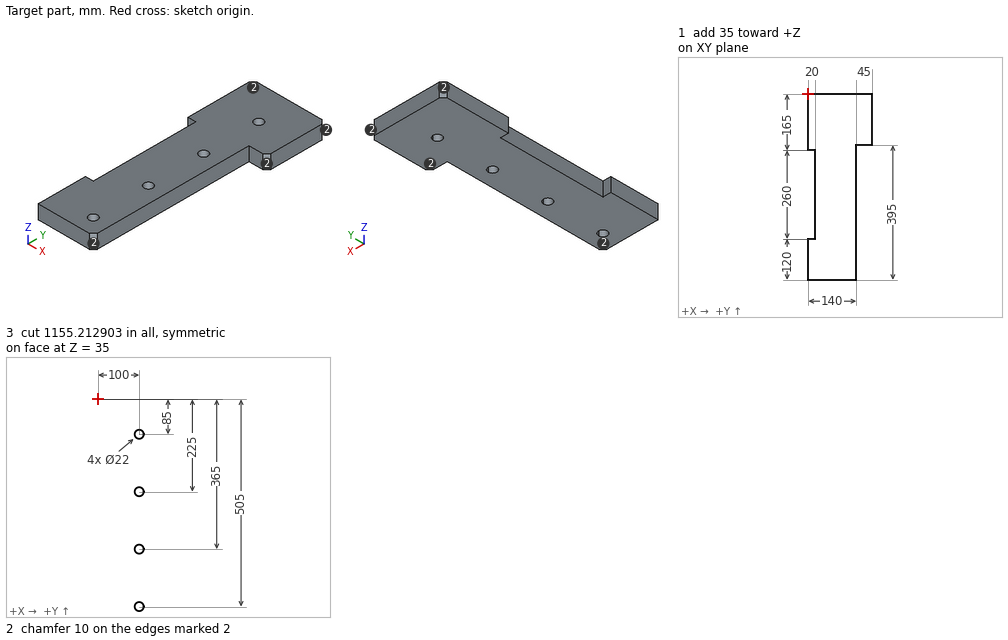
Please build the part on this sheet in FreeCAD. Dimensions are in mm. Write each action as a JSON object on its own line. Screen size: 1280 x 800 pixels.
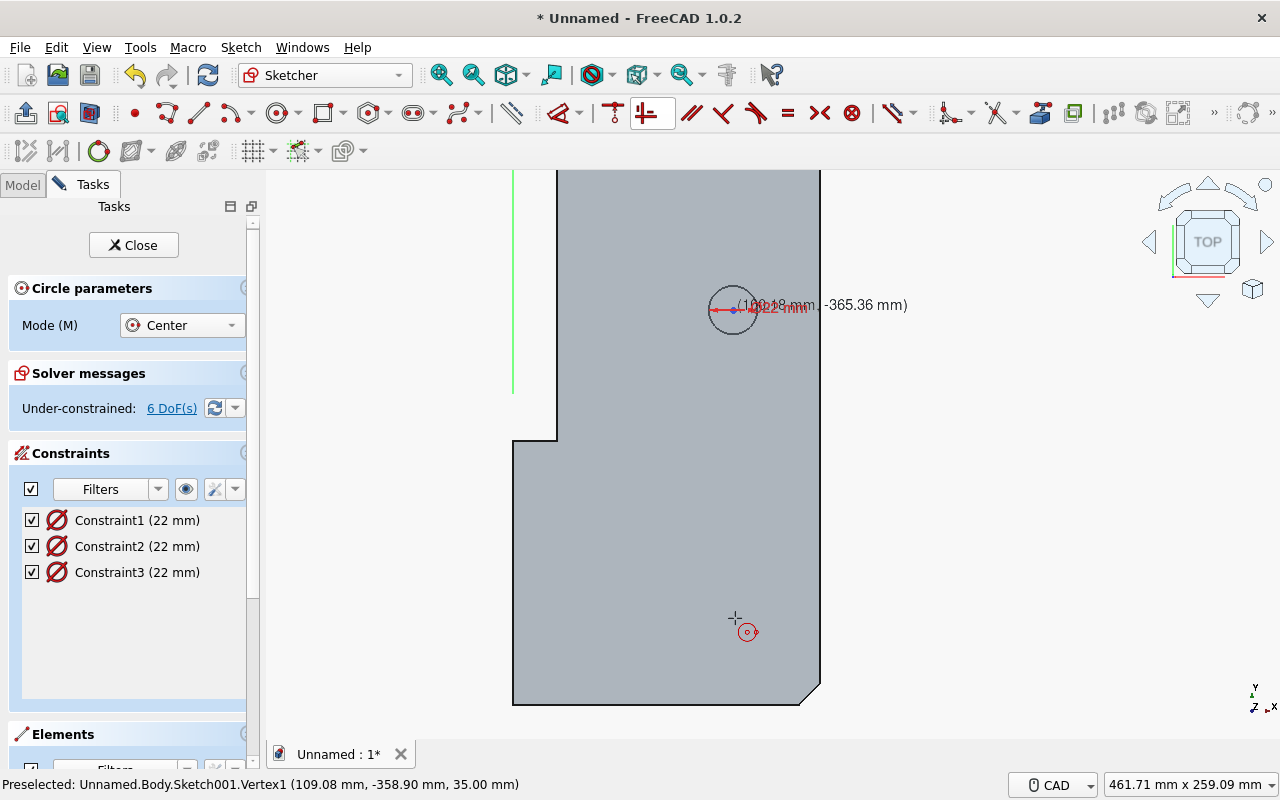
{"action": "left_click", "coordinate": [733, 617]}
{"action": "mouse_move", "coordinate": [750, 600]}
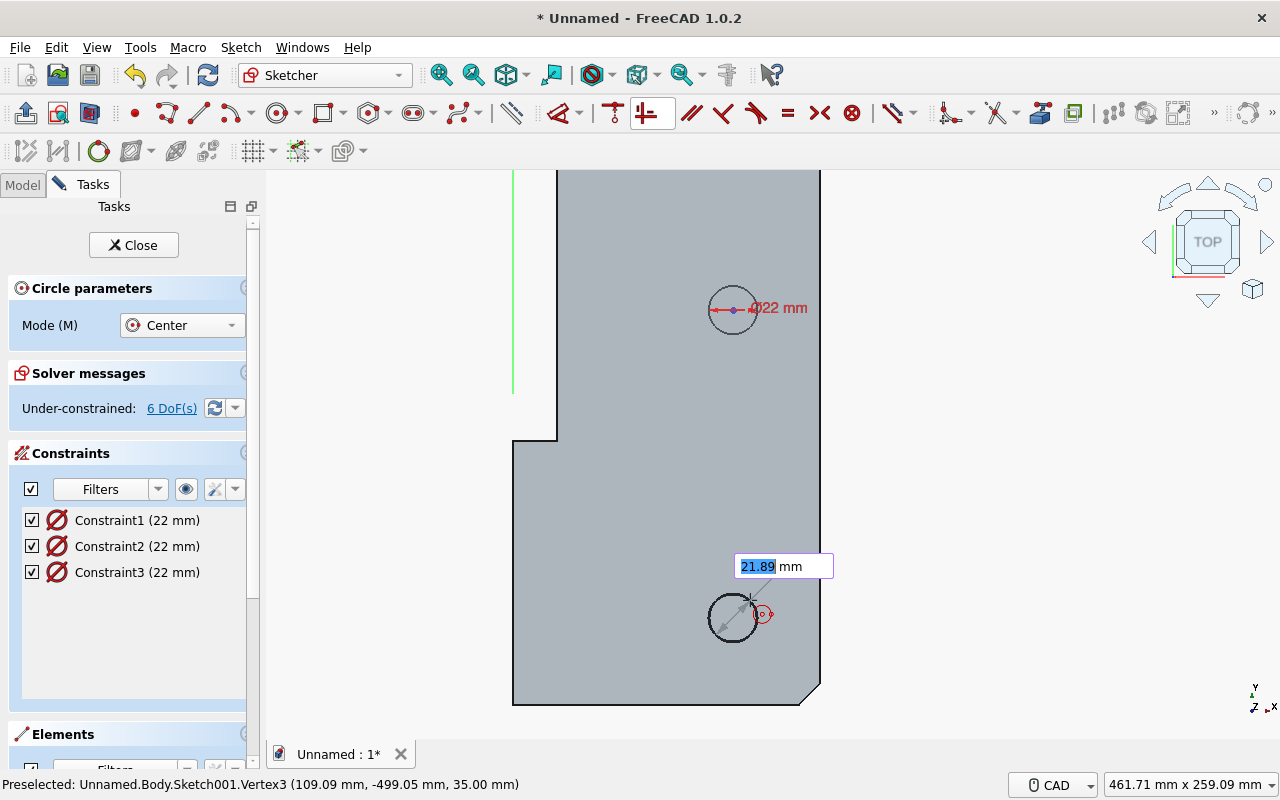
{"action": "type", "text": "22"}
{"action": "key", "text": "Return"}
{"action": "key", "text": "Escape"}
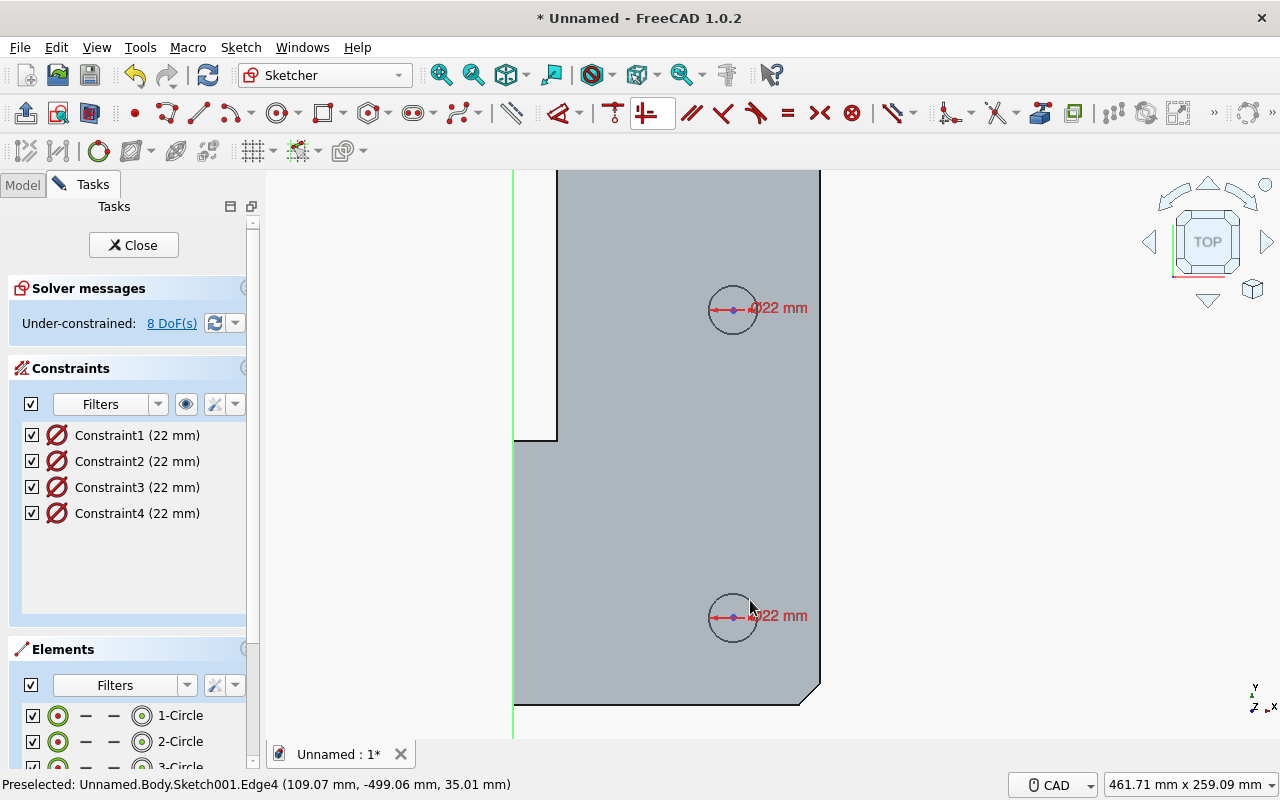
{"action": "scroll", "coordinate": [735, 618], "scroll_direction": "down", "scroll_amount": 6}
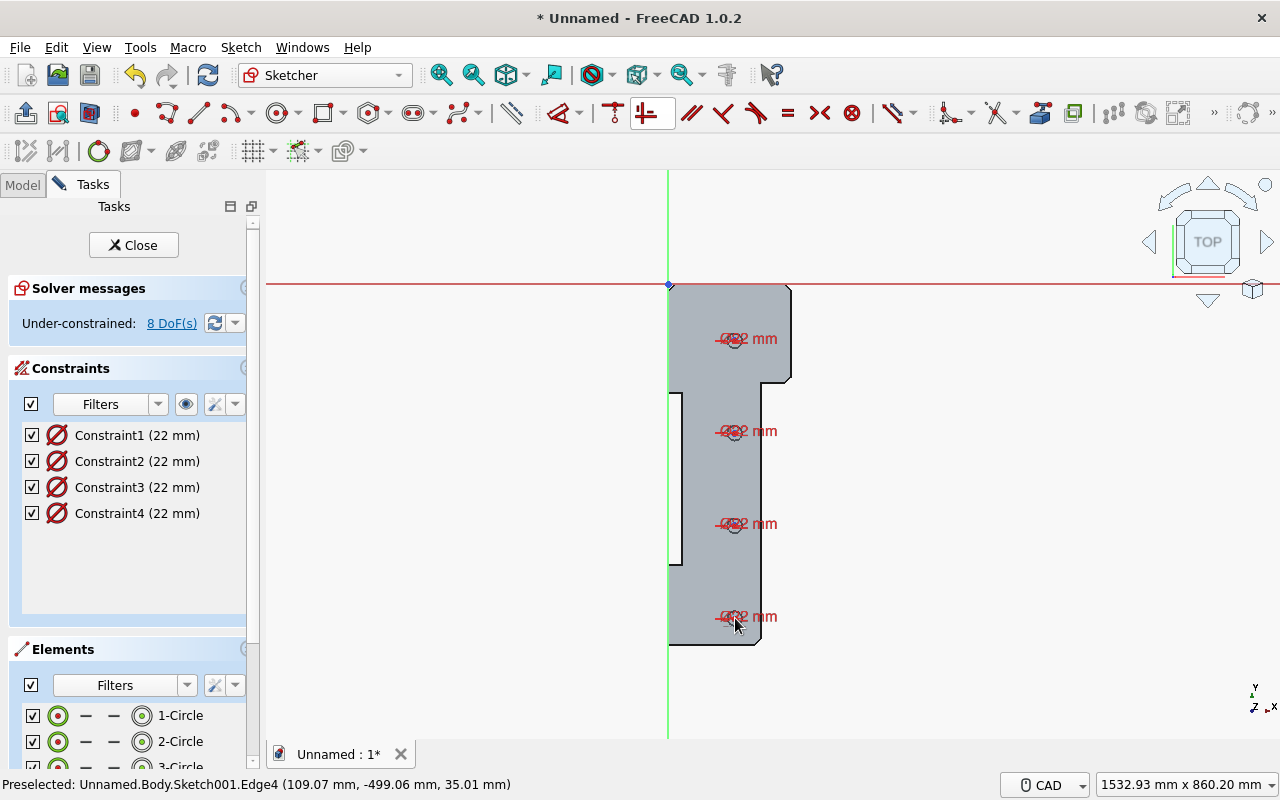
{"action": "left_click", "coordinate": [735, 341]}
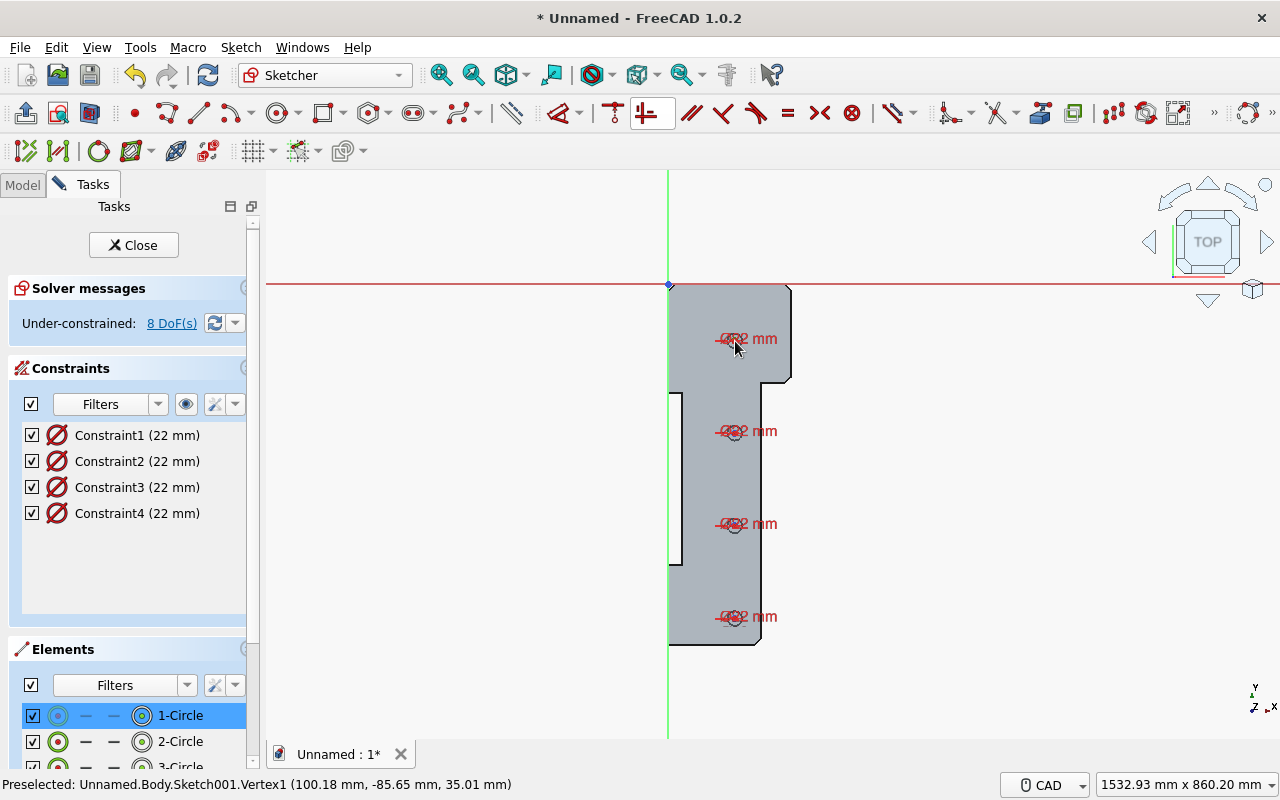
{"action": "left_click", "coordinate": [735, 433]}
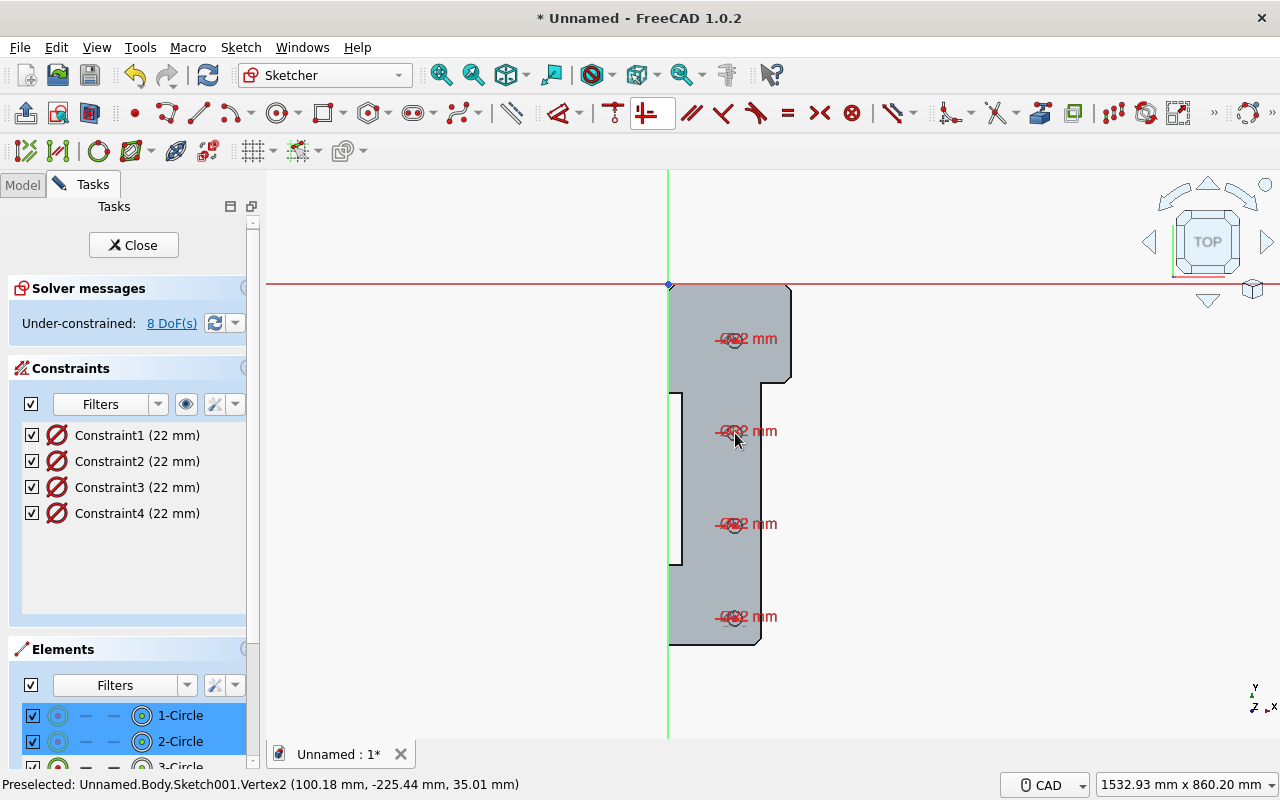
{"action": "left_click", "coordinate": [670, 114]}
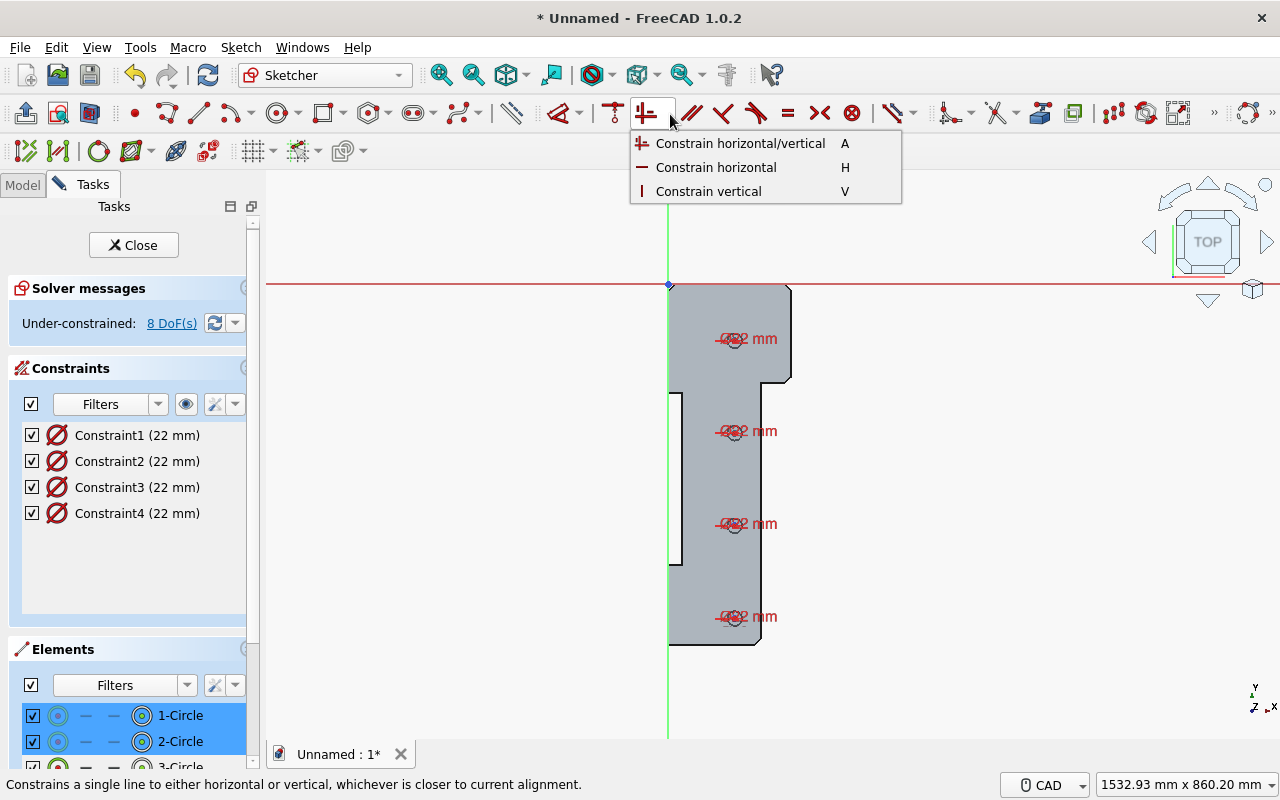
{"action": "left_click", "coordinate": [766, 191]}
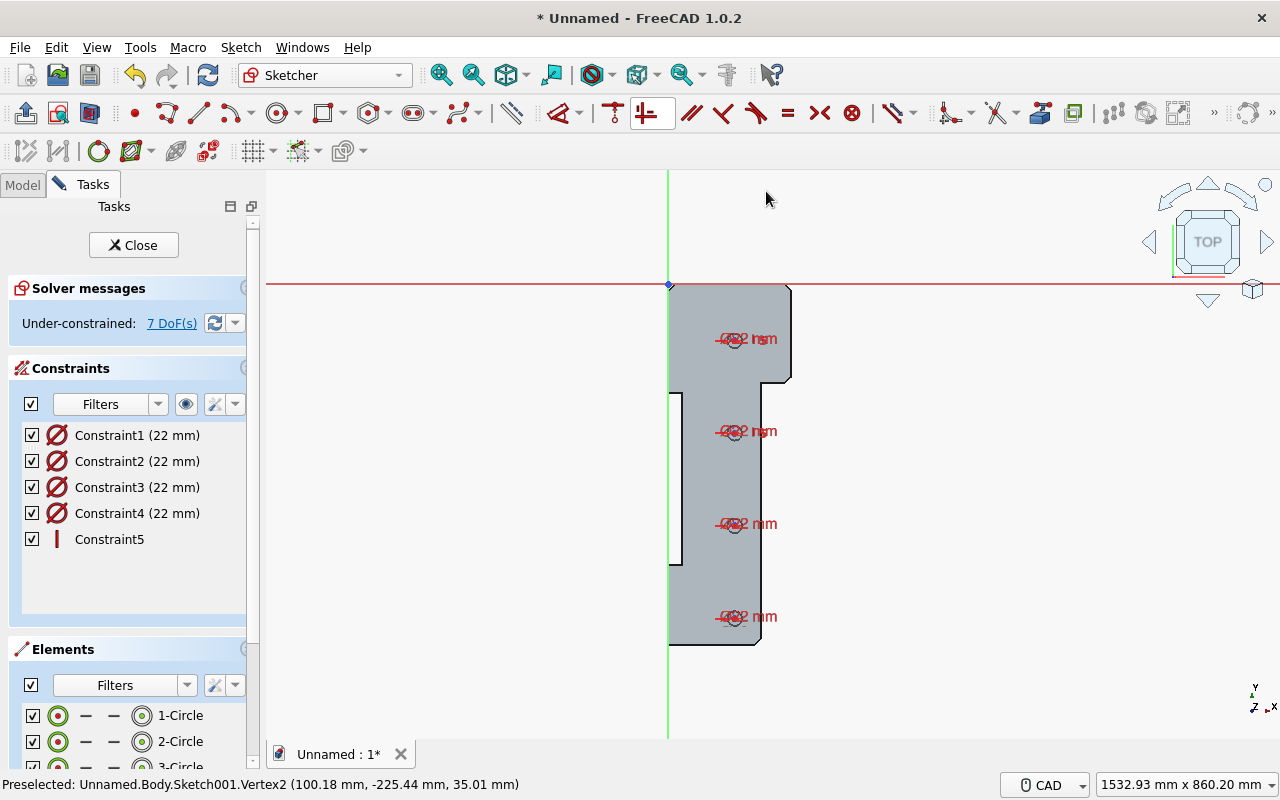
{"action": "left_click", "coordinate": [735, 433]}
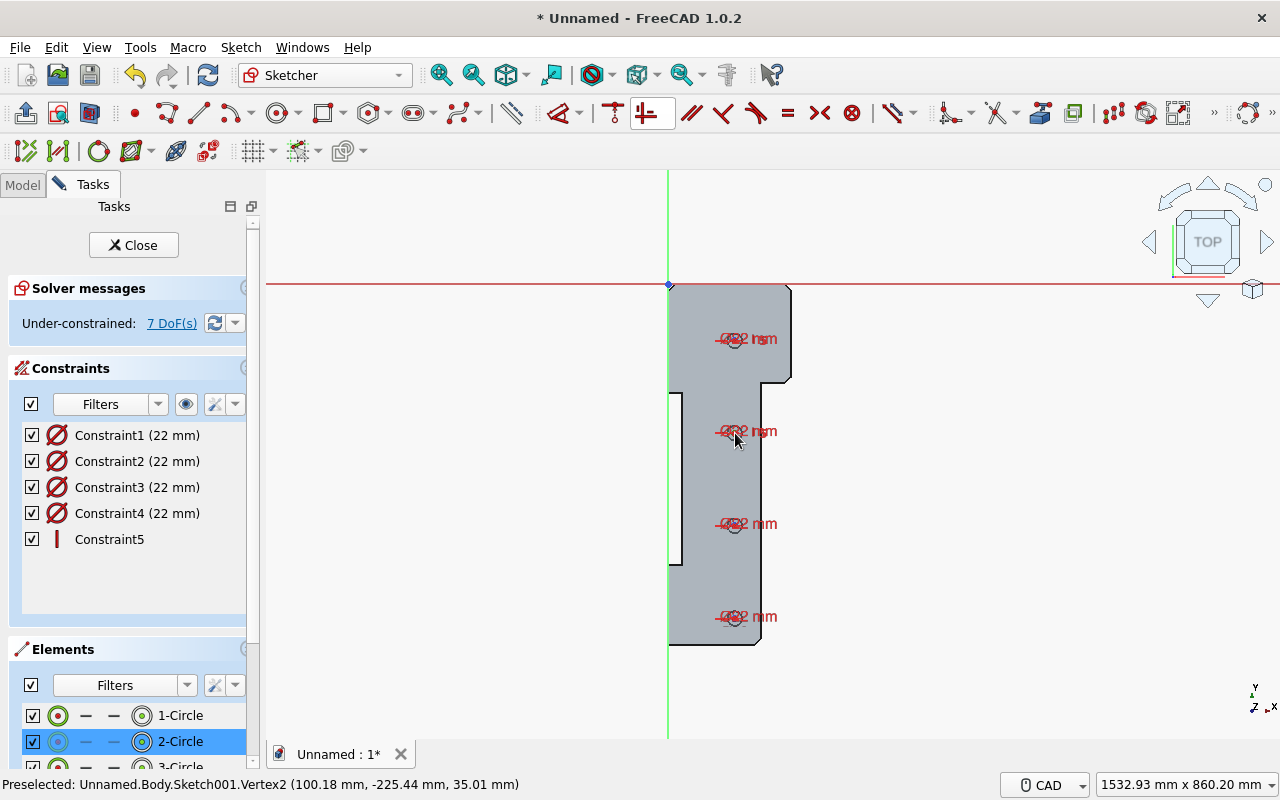
{"action": "left_click", "coordinate": [735, 526]}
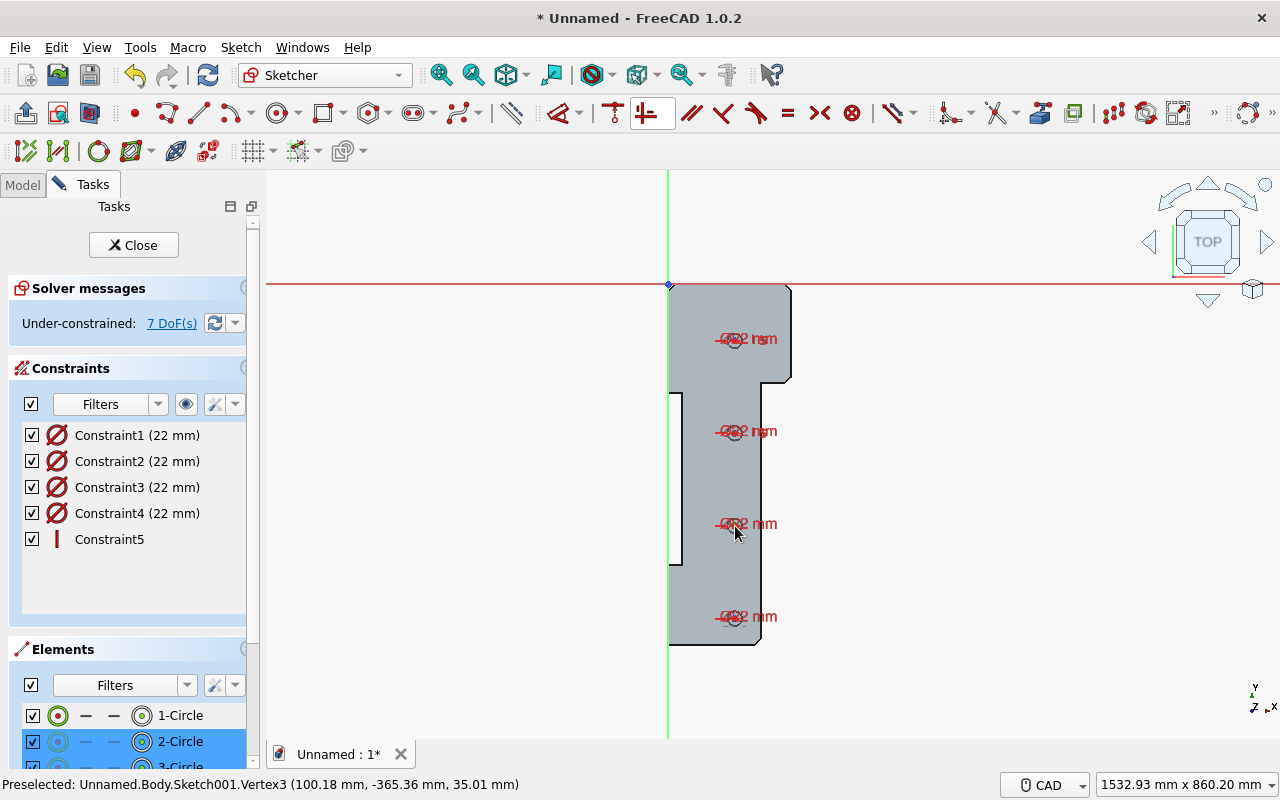
{"action": "left_click", "coordinate": [670, 114]}